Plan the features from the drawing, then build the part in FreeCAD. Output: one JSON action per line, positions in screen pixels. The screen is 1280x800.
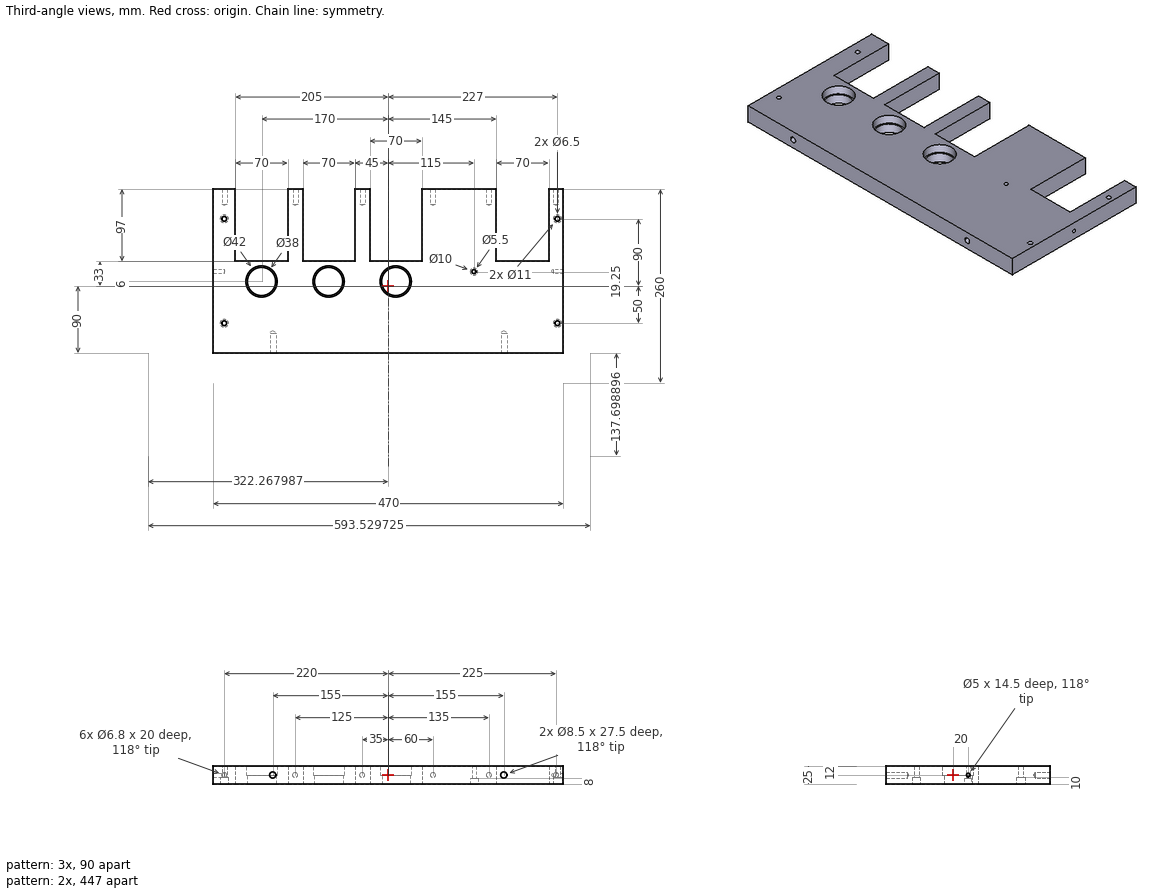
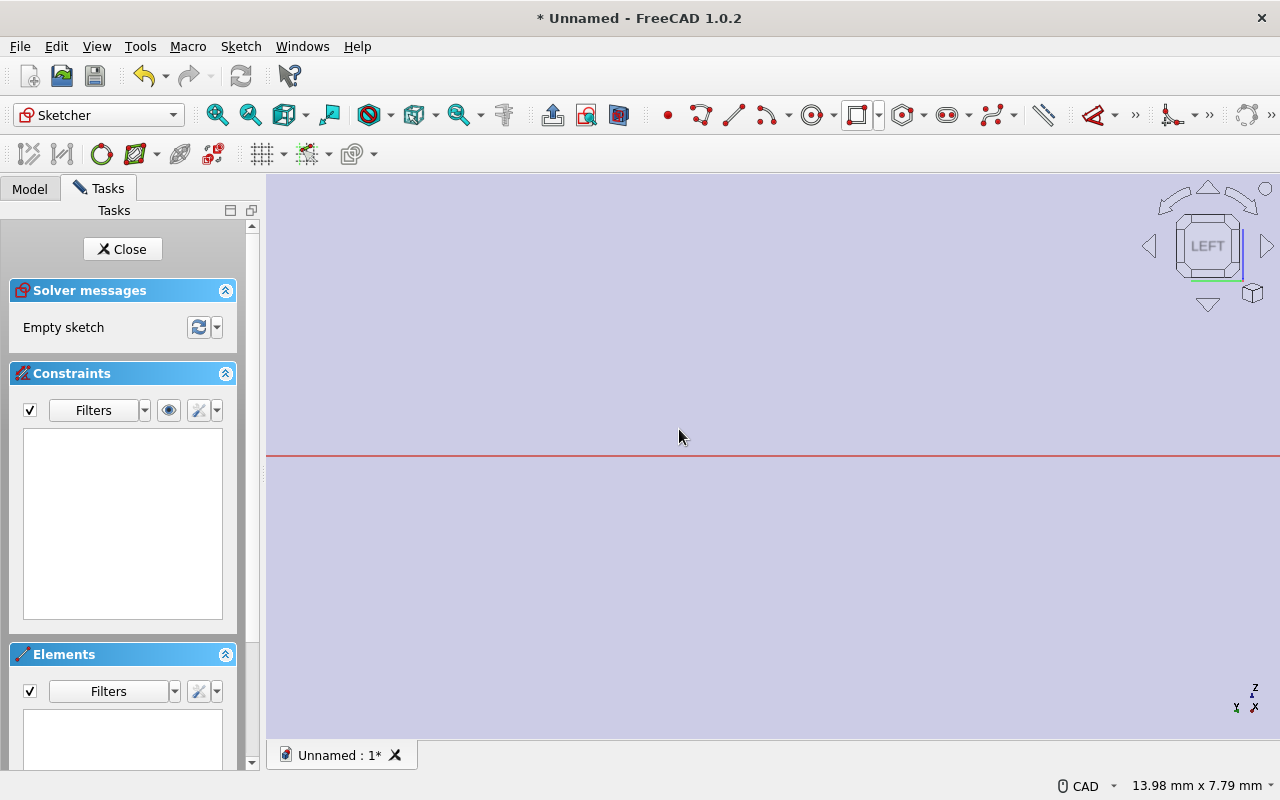
{"action": "left_click", "coordinate": [812, 116]}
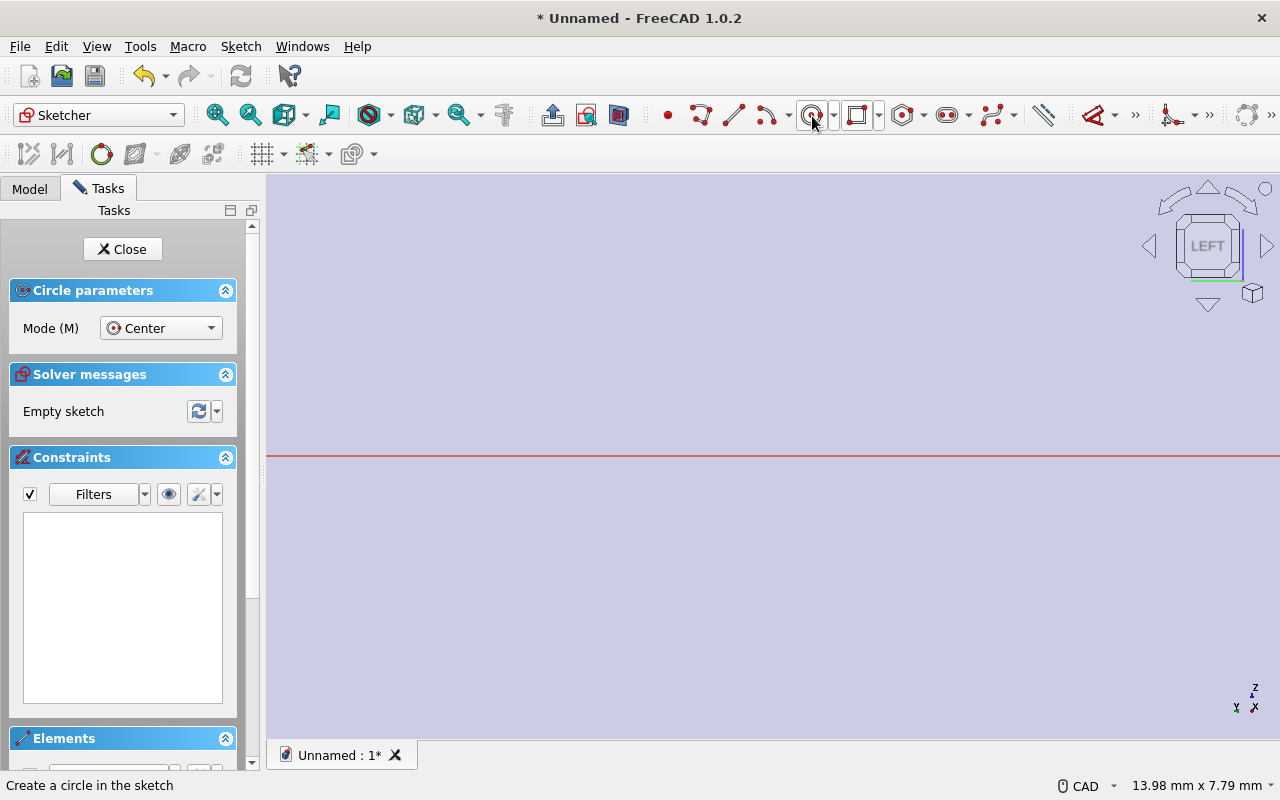
{"action": "left_click", "coordinate": [705, 456]}
{"action": "mouse_move", "coordinate": [833, 328]}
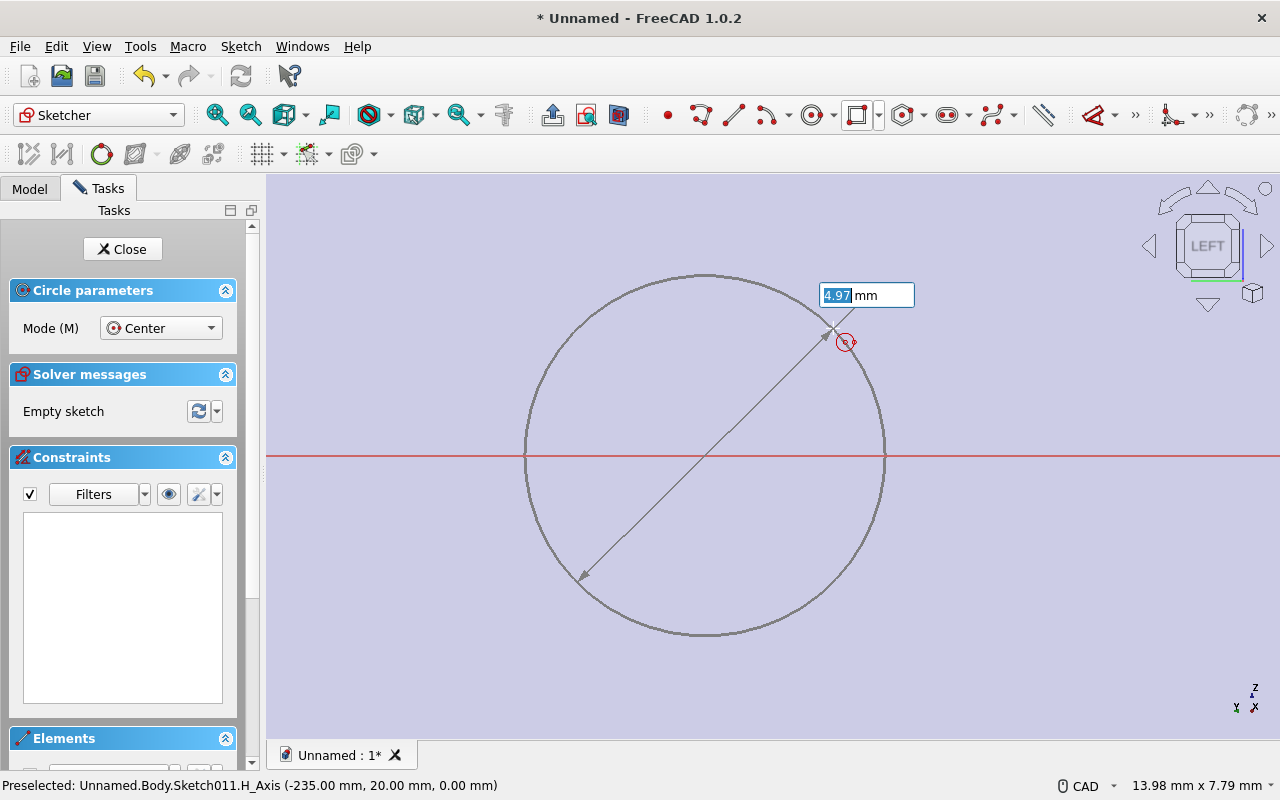
{"action": "type", "text": "5"}
{"action": "key", "text": "Return"}
{"action": "key", "text": "Escape"}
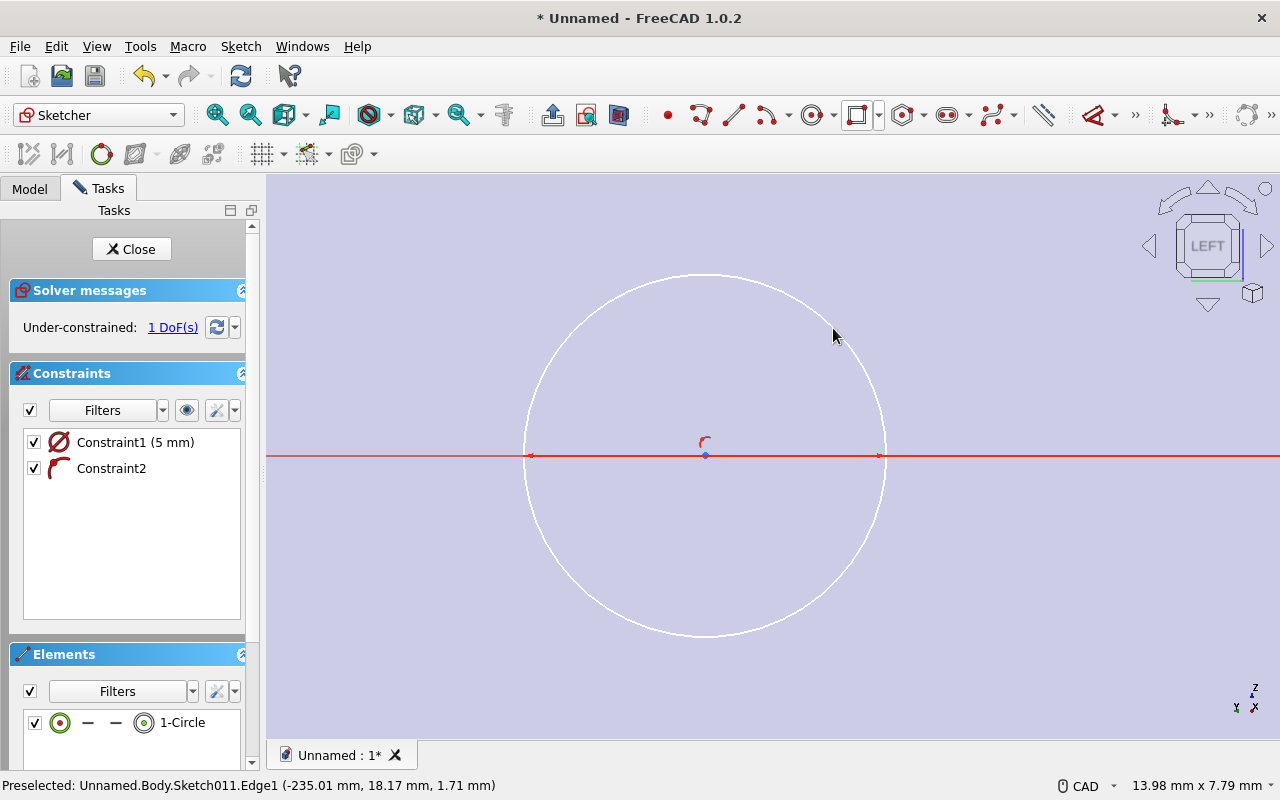
{"action": "left_click", "coordinate": [1092, 116]}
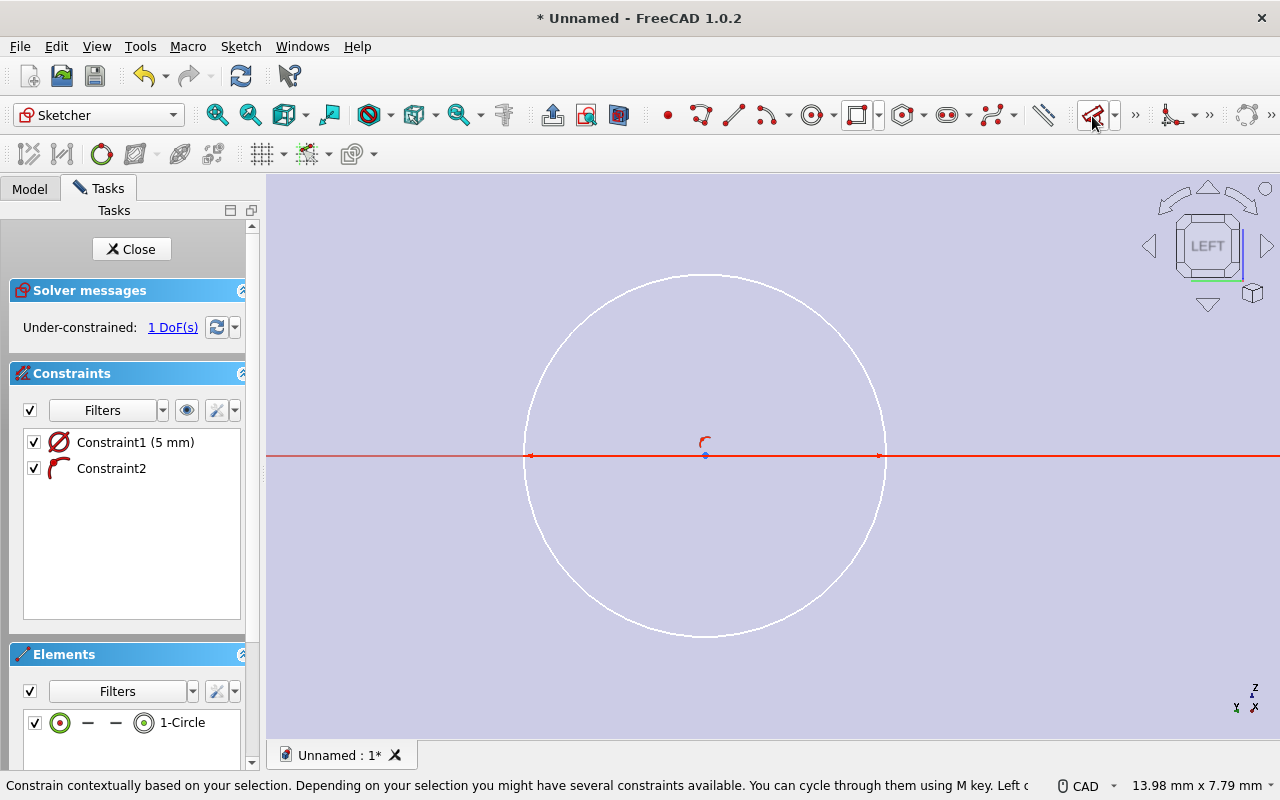
{"action": "left_click", "coordinate": [705, 456]}
{"action": "left_click", "coordinate": [910, 490]}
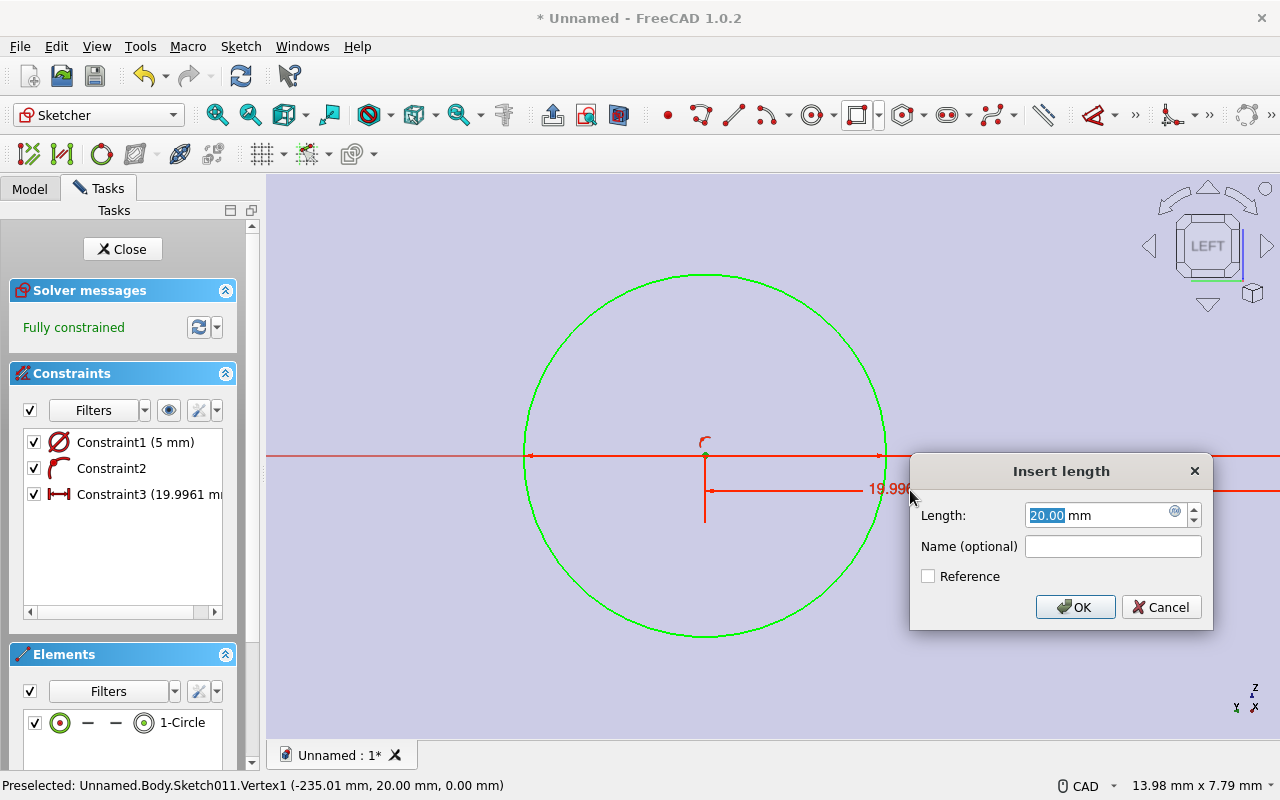
{"action": "type", "text": "20"}
{"action": "key", "text": "Return"}
{"action": "key", "text": "Escape"}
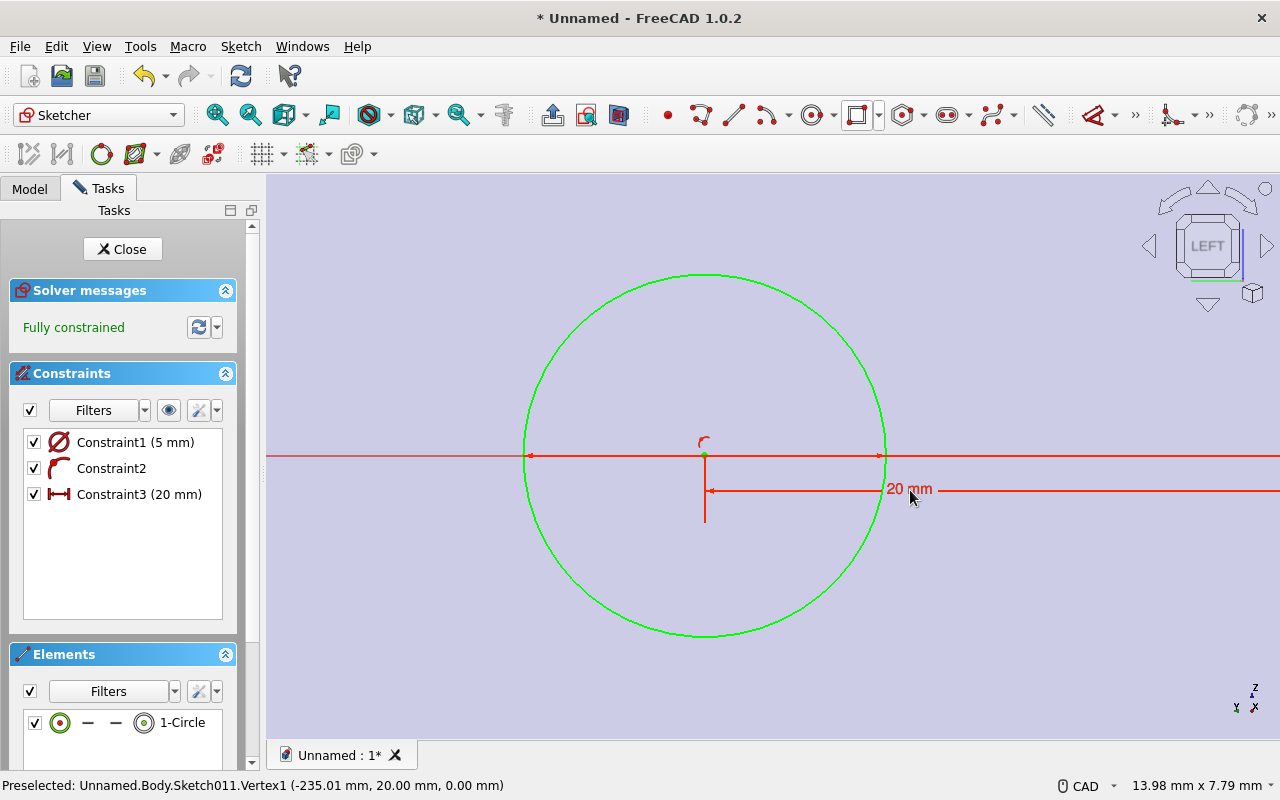
{"action": "left_click", "coordinate": [123, 249]}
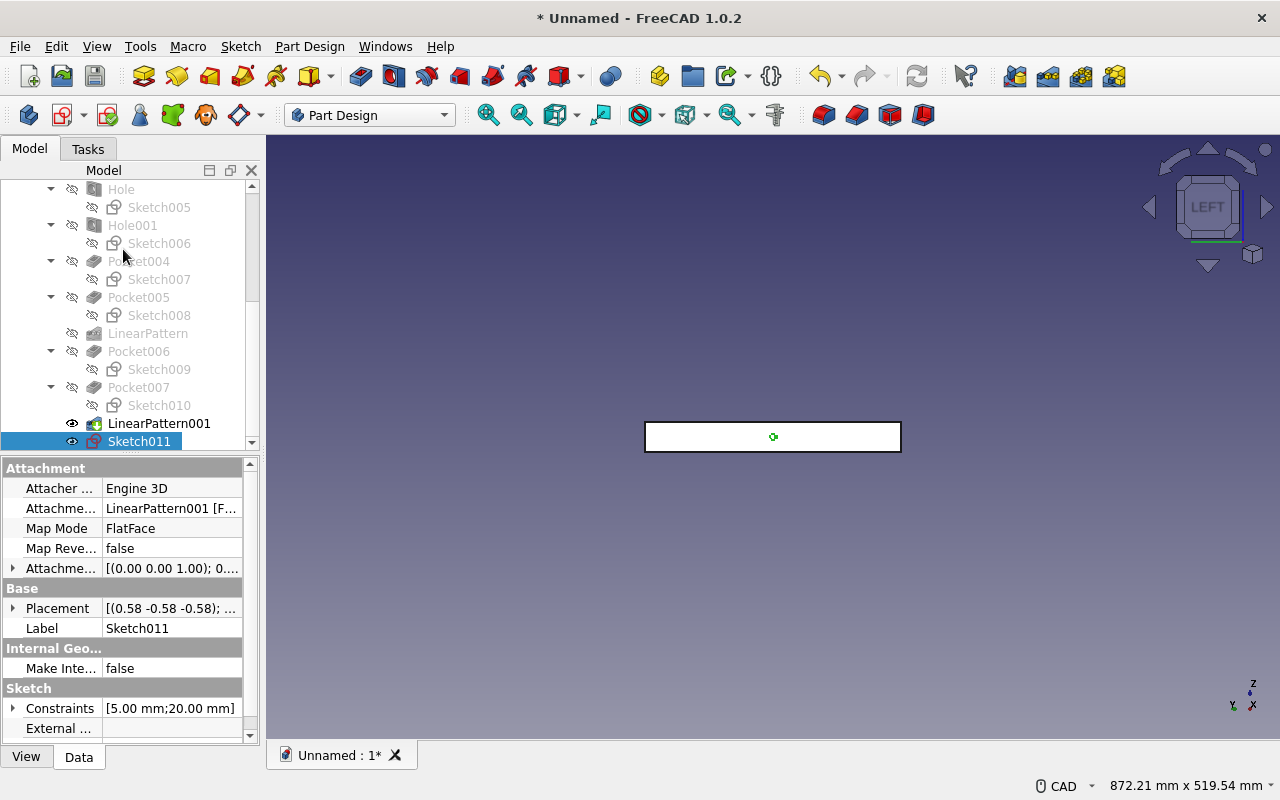
{"action": "left_click", "coordinate": [394, 76]}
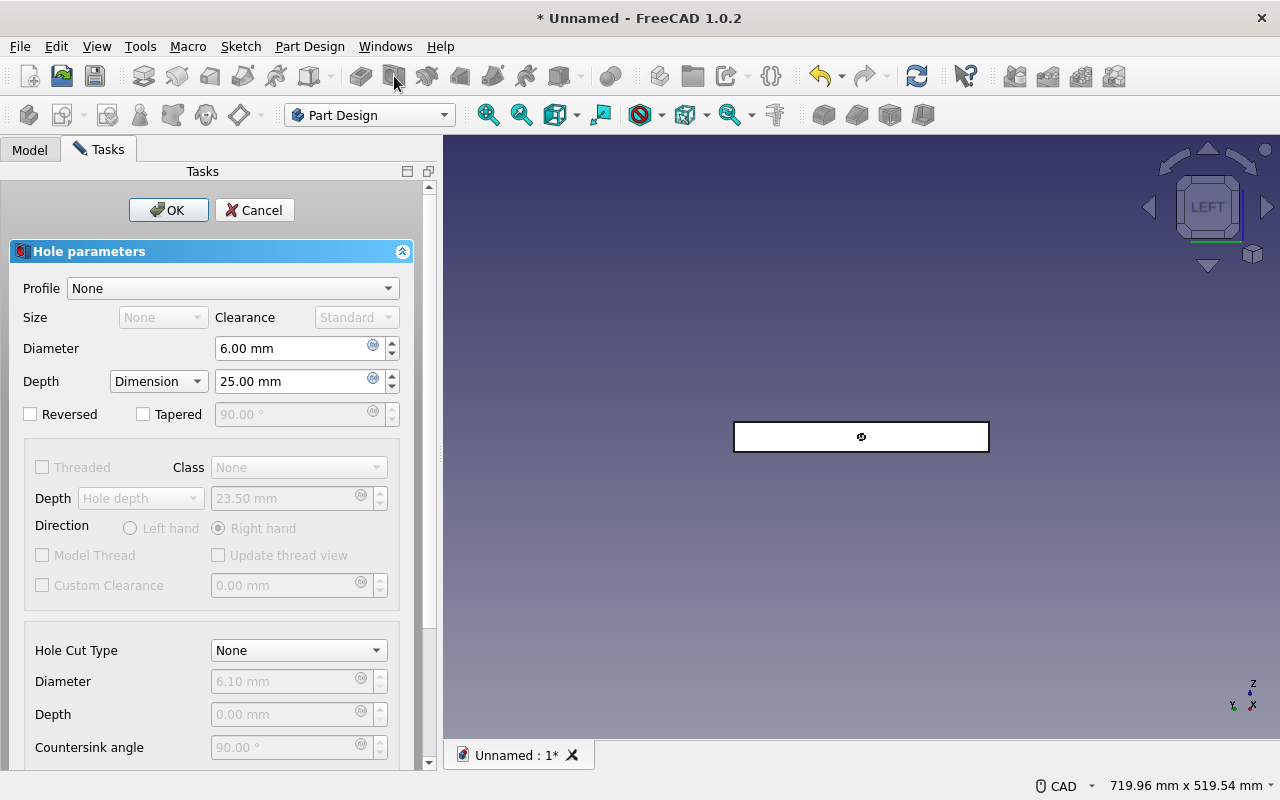
{"action": "triple_click", "coordinate": [300, 348]}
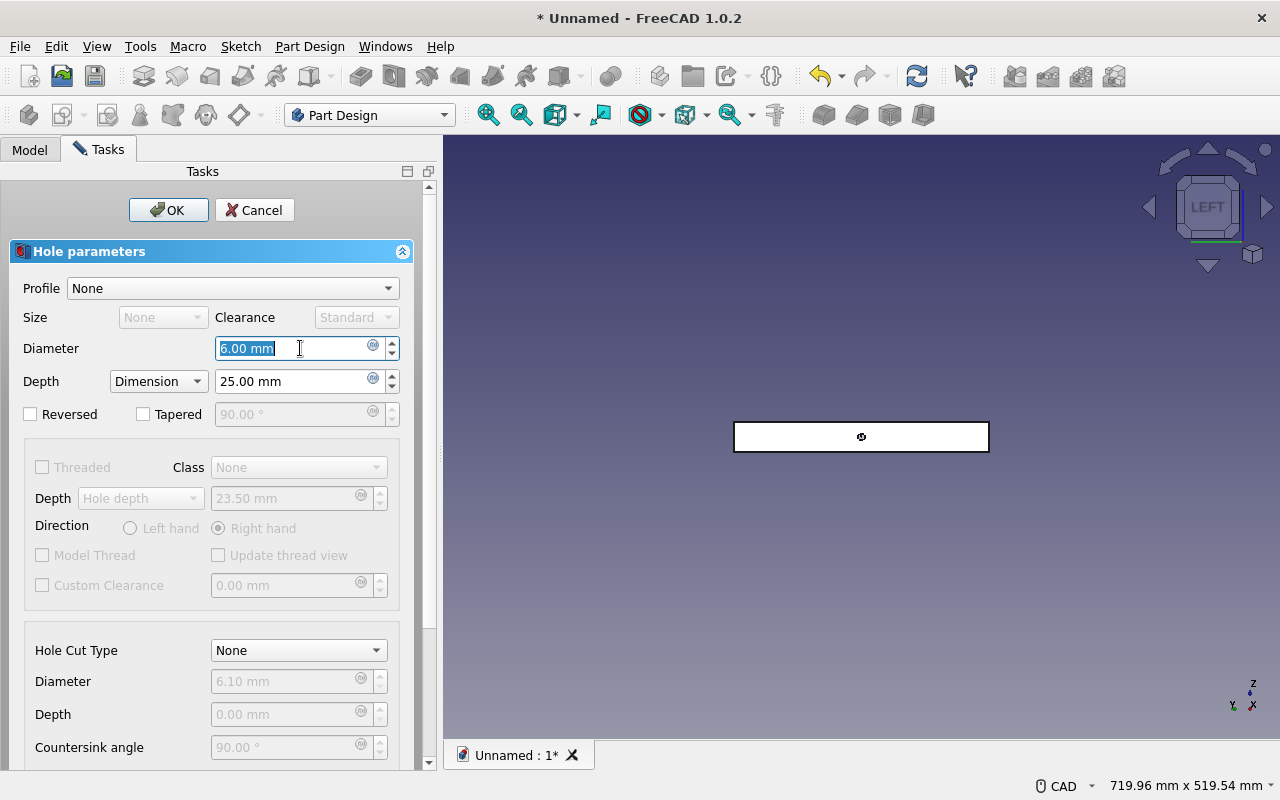
{"action": "type", "text": "5"}
{"action": "key", "text": "Tab"}